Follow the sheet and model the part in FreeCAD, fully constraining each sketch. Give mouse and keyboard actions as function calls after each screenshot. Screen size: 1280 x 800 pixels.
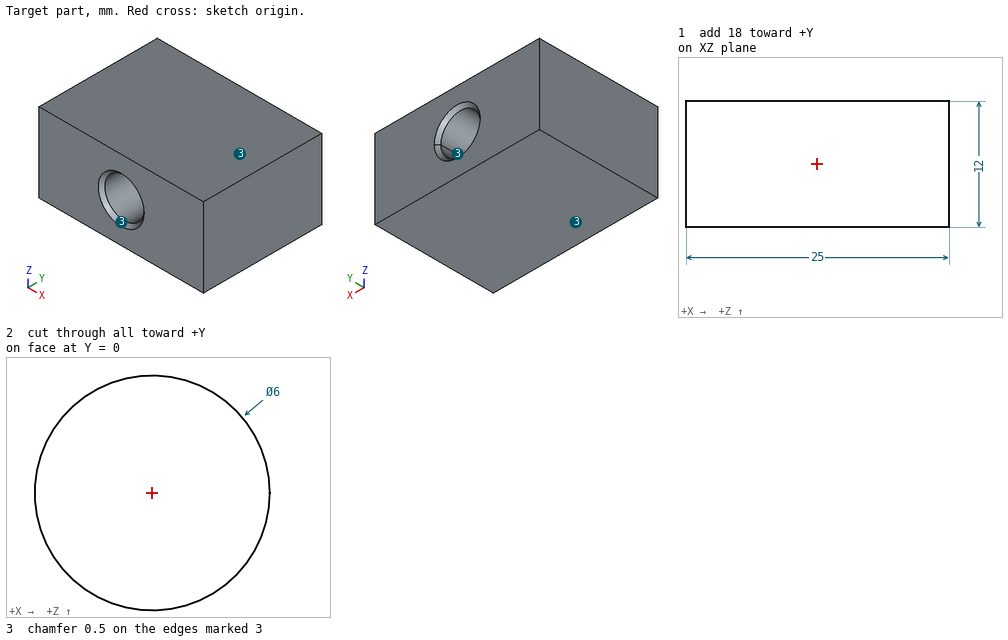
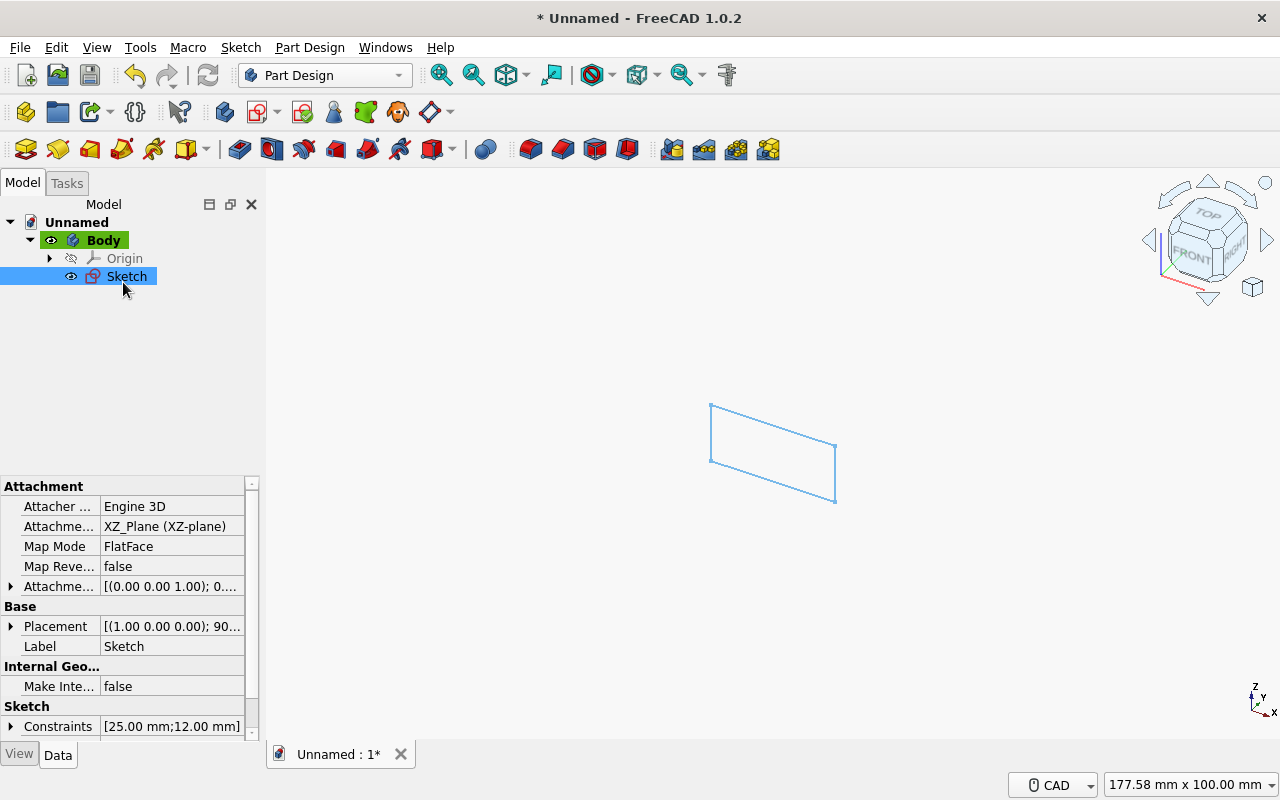
click(26, 150)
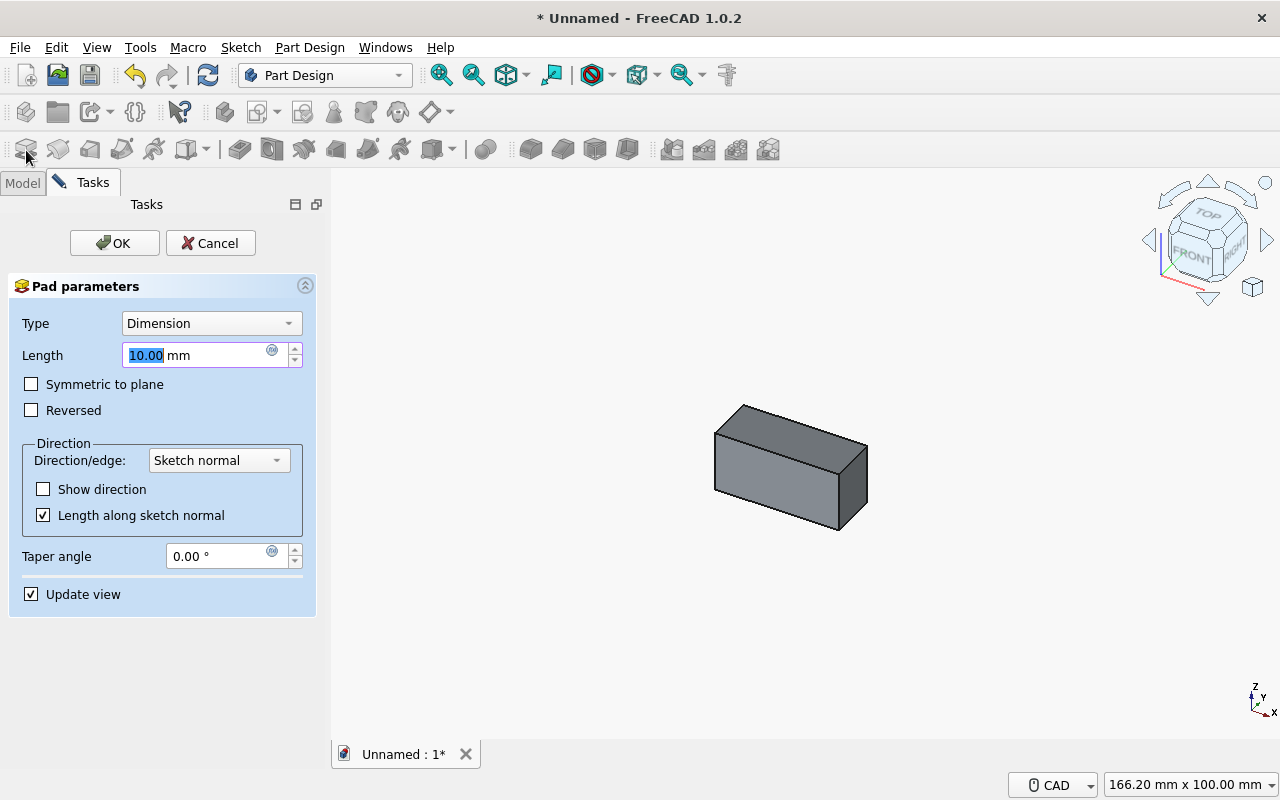
text(18)
key(Tab)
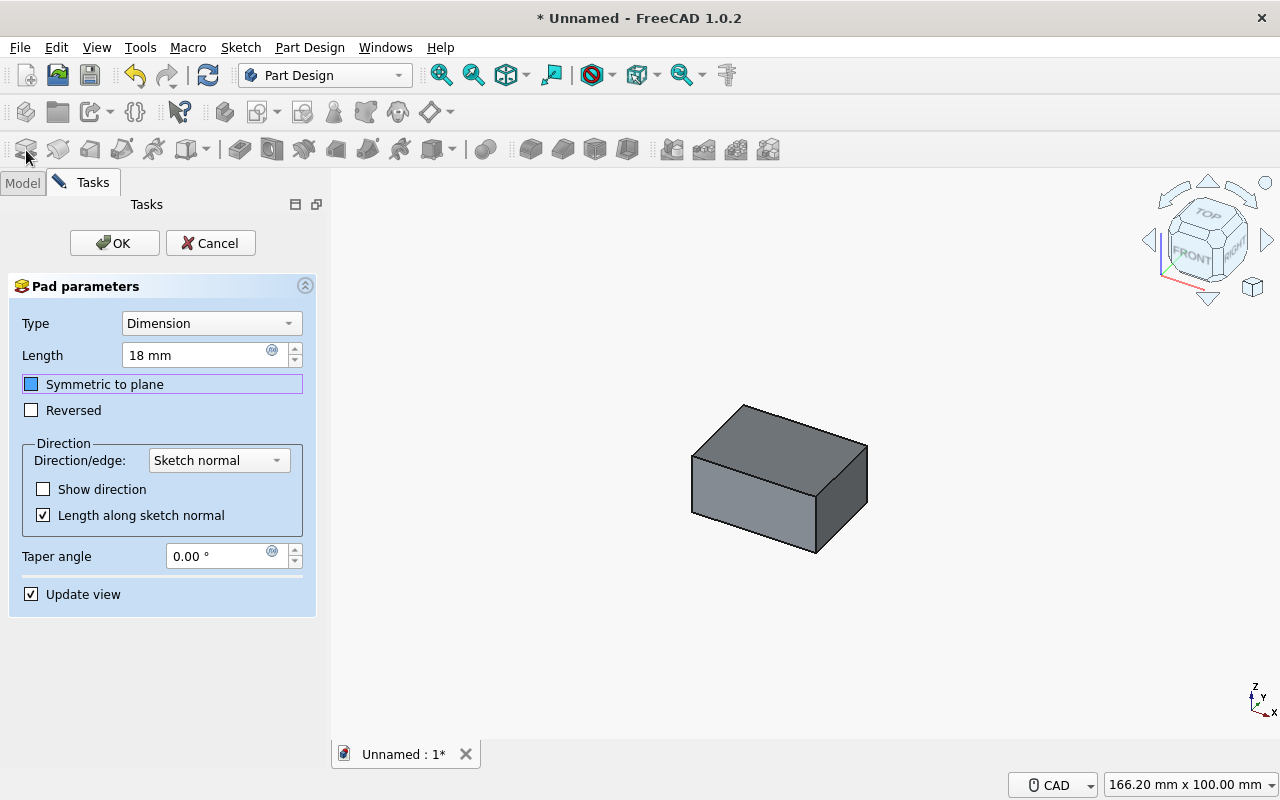
click(30, 410)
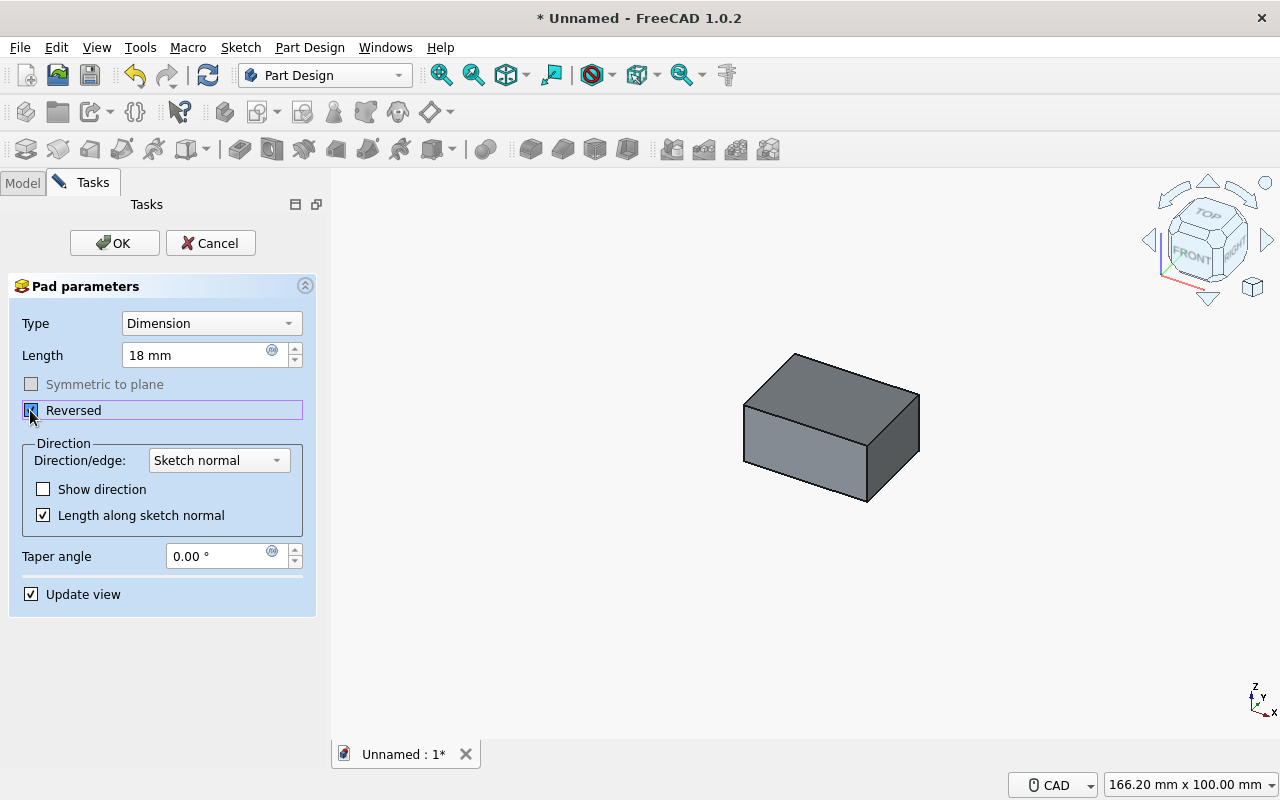
click(115, 243)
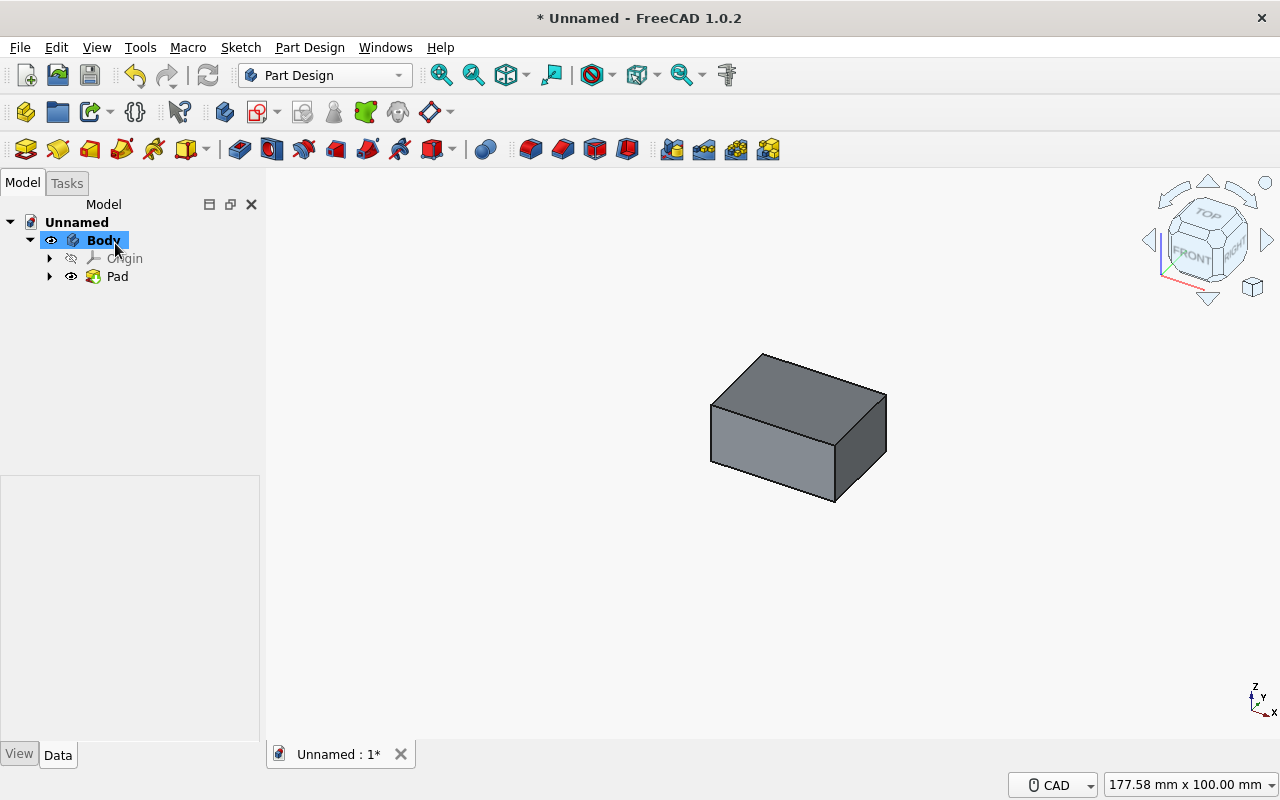
click(442, 76)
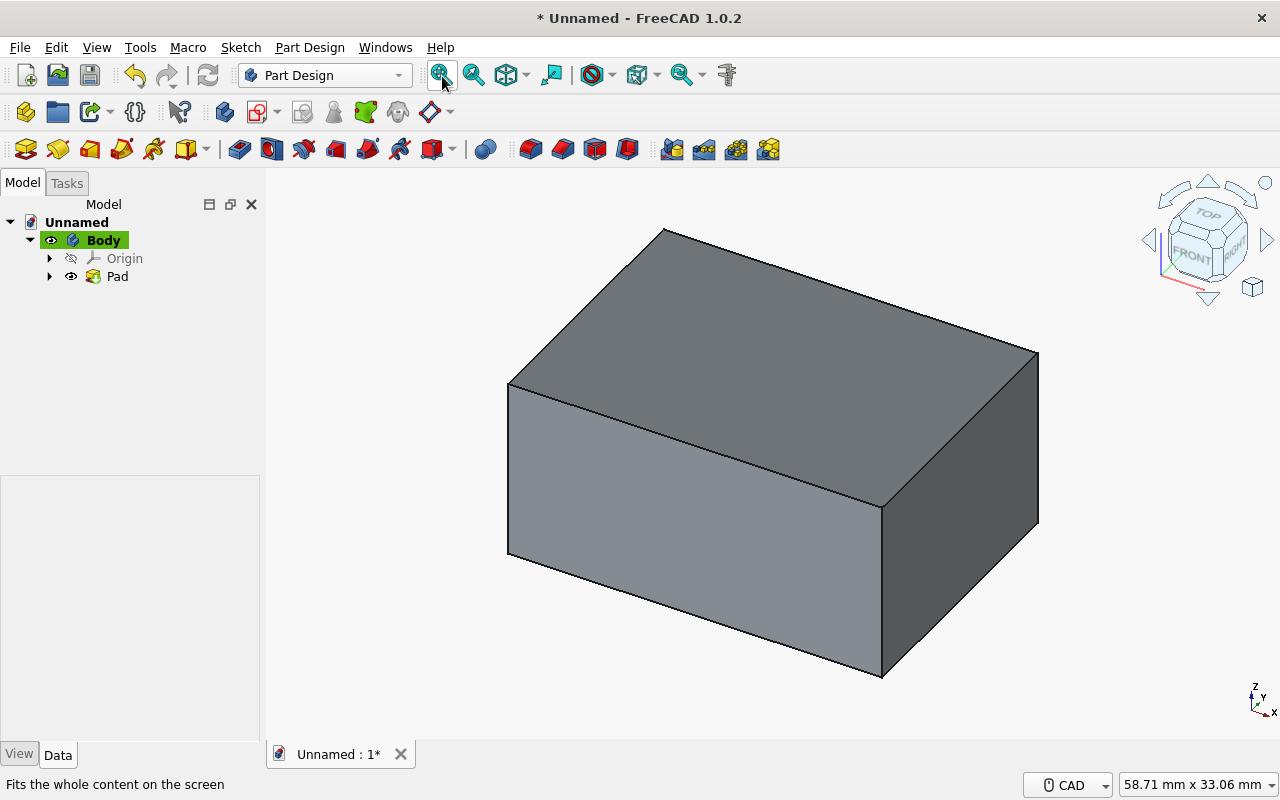
click(749, 547)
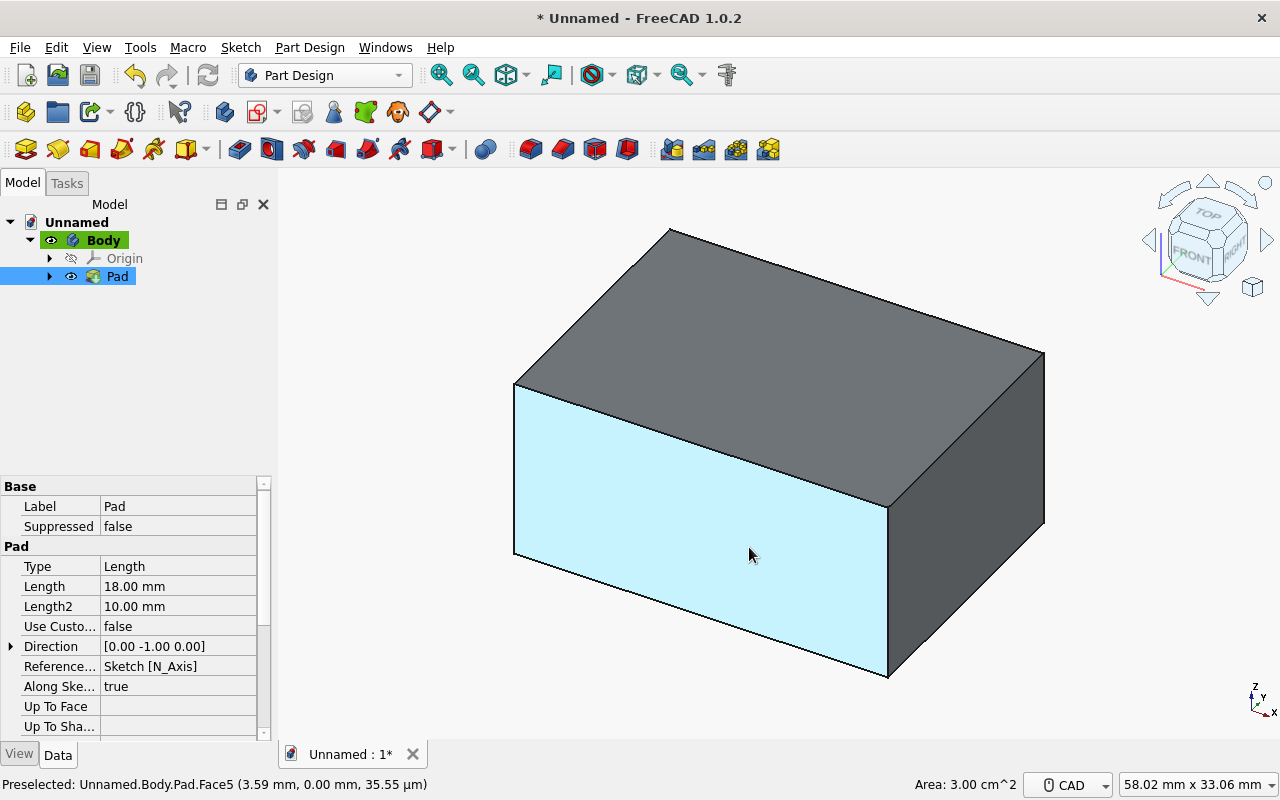
click(258, 112)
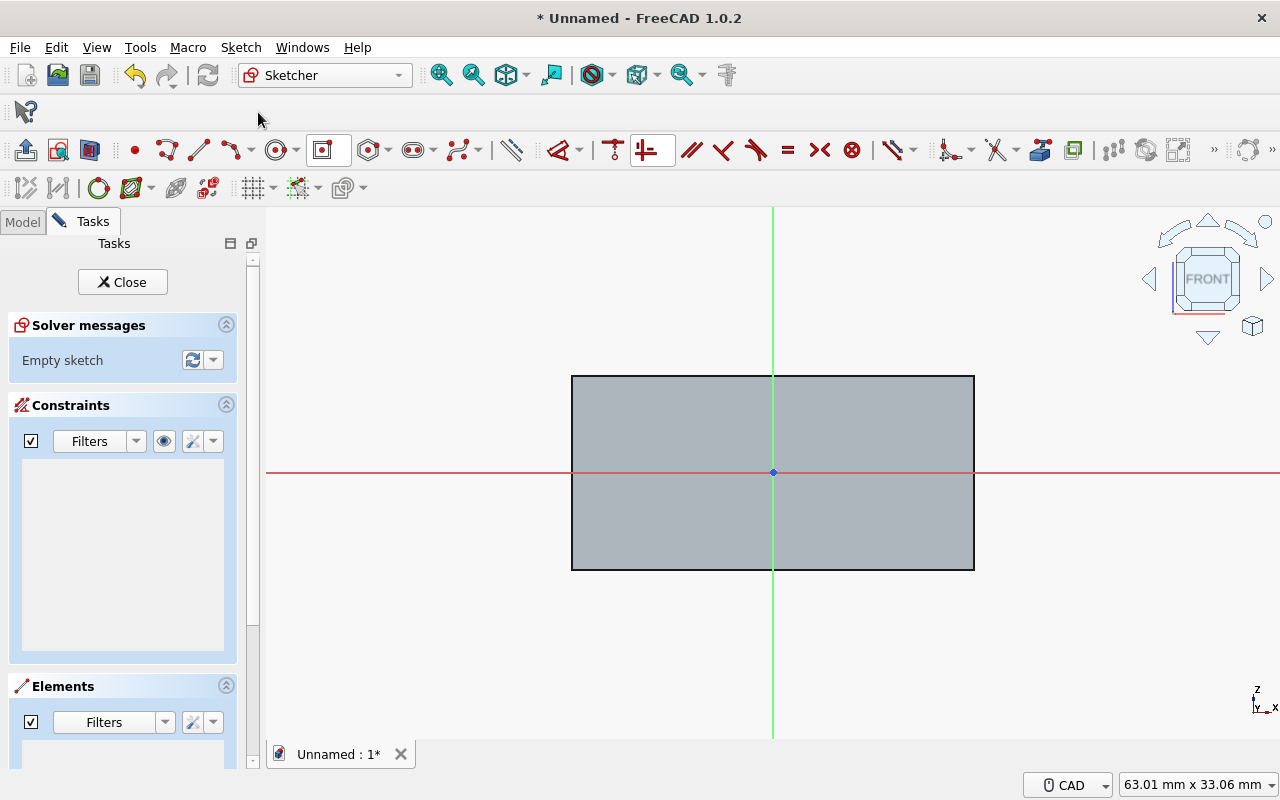
scroll(803, 473, up, 6)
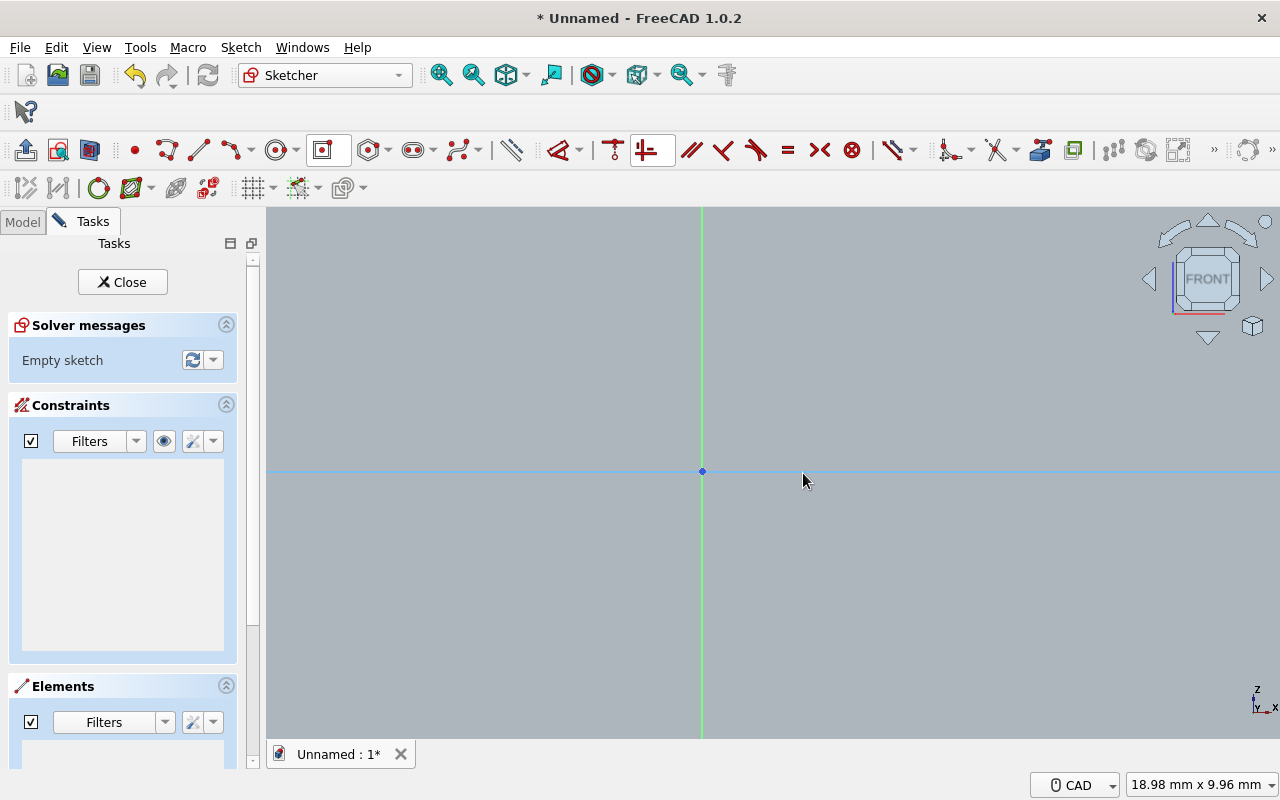
click(276, 150)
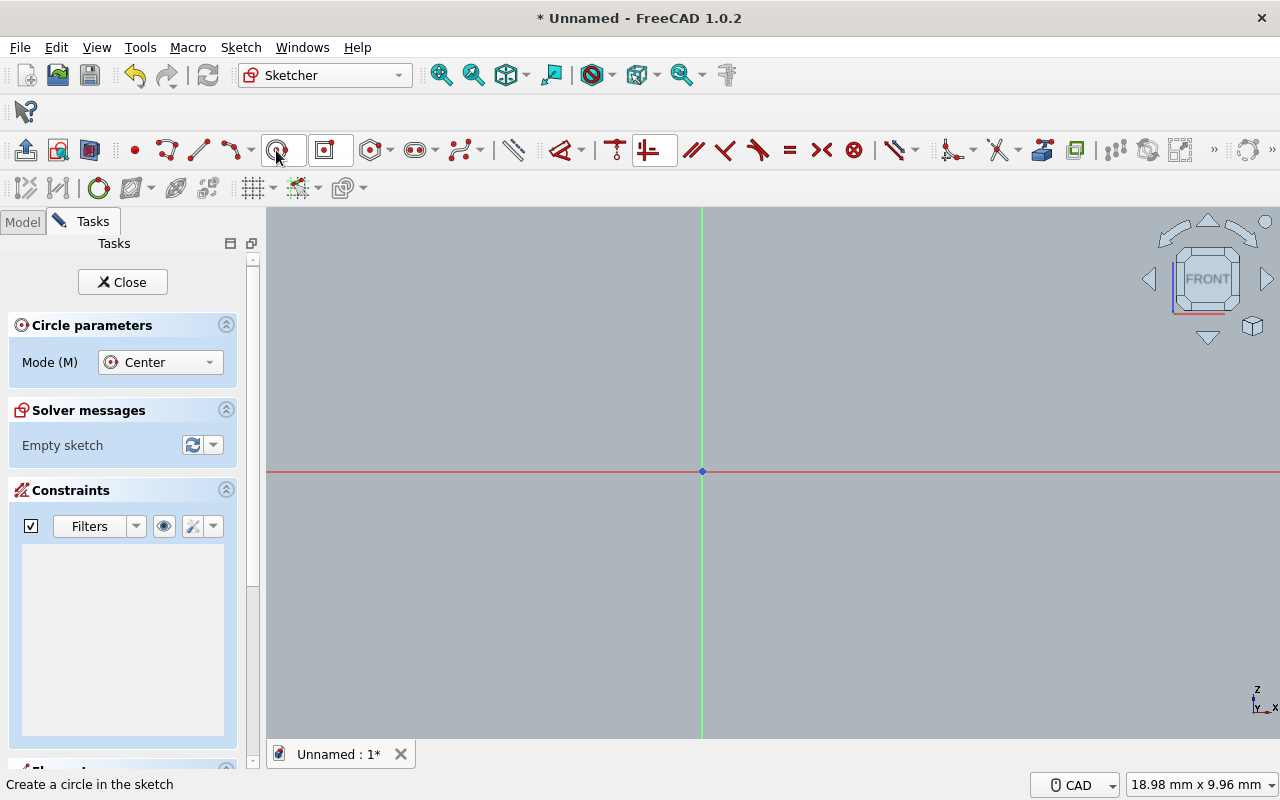
click(702, 472)
move(816, 359)